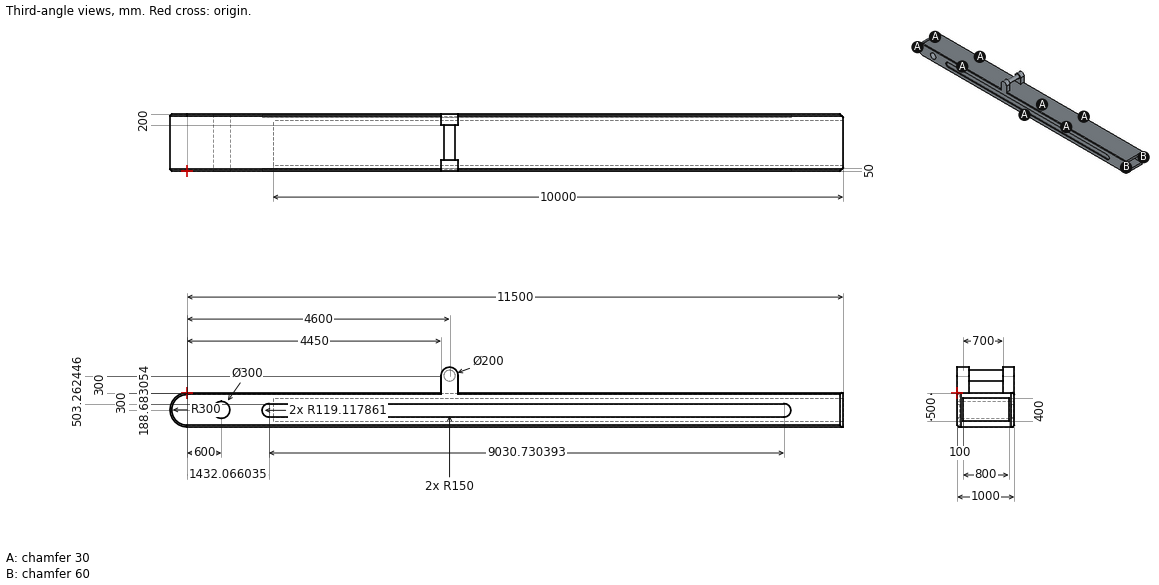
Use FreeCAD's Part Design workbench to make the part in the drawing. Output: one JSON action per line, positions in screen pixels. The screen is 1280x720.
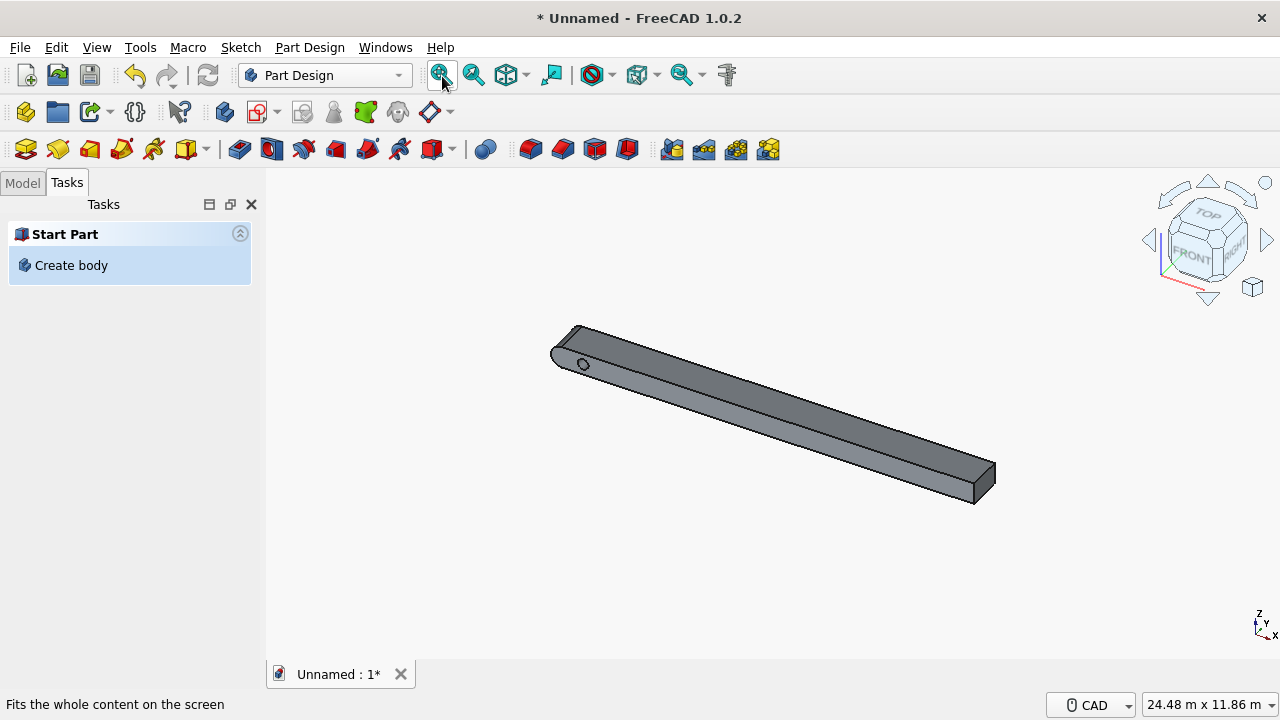
{"action": "key", "text": "4"}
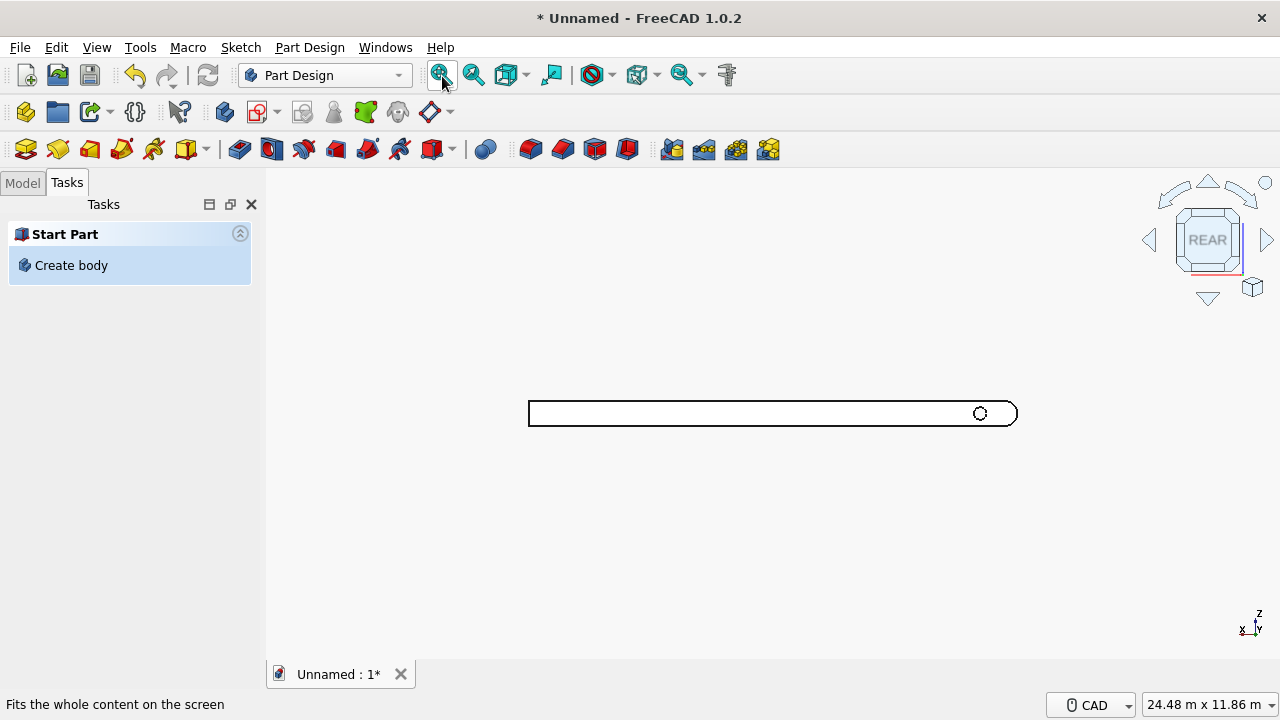
{"action": "left_click", "coordinate": [564, 412]}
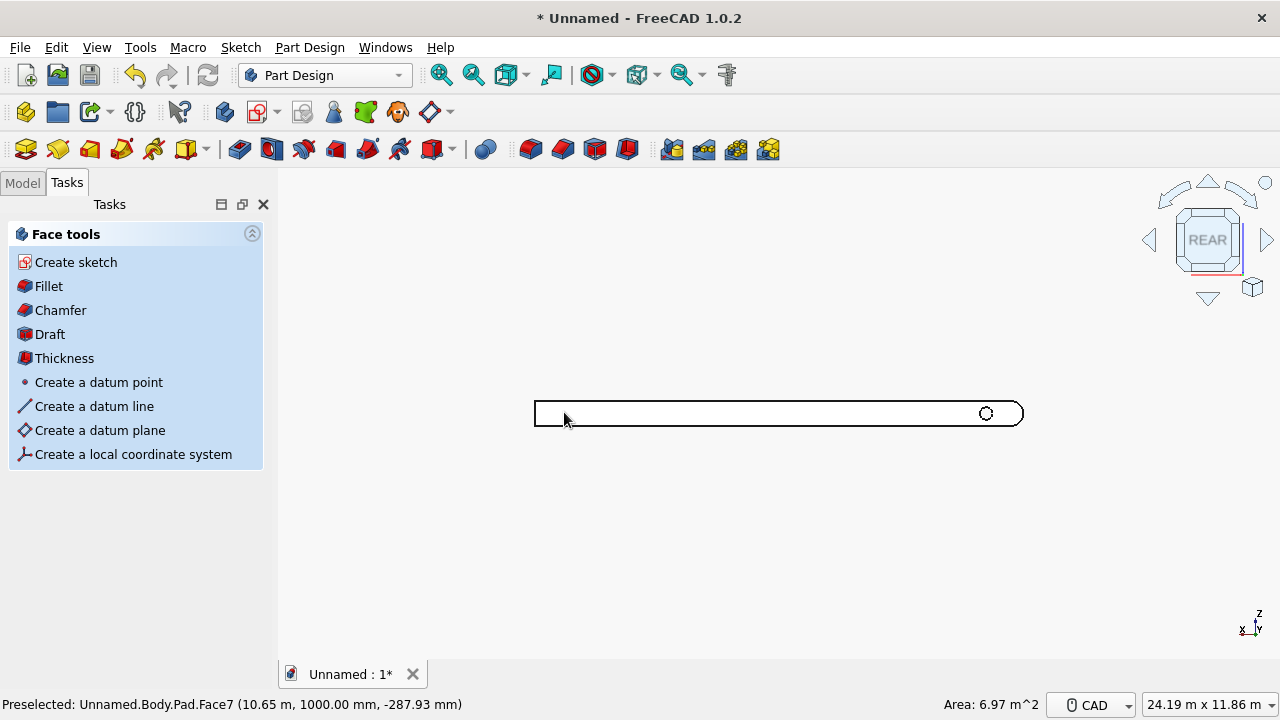
{"action": "left_click", "coordinate": [258, 112]}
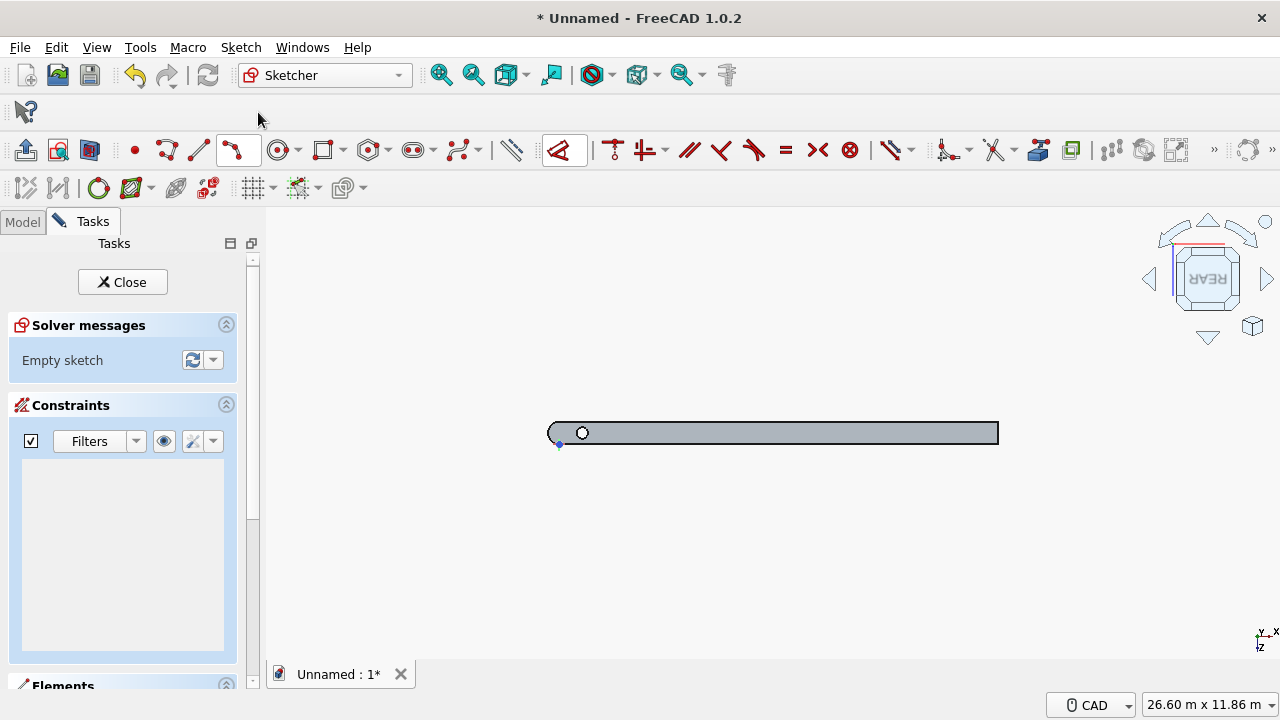
{"action": "scroll", "coordinate": [739, 448], "scroll_direction": "up", "scroll_amount": 11}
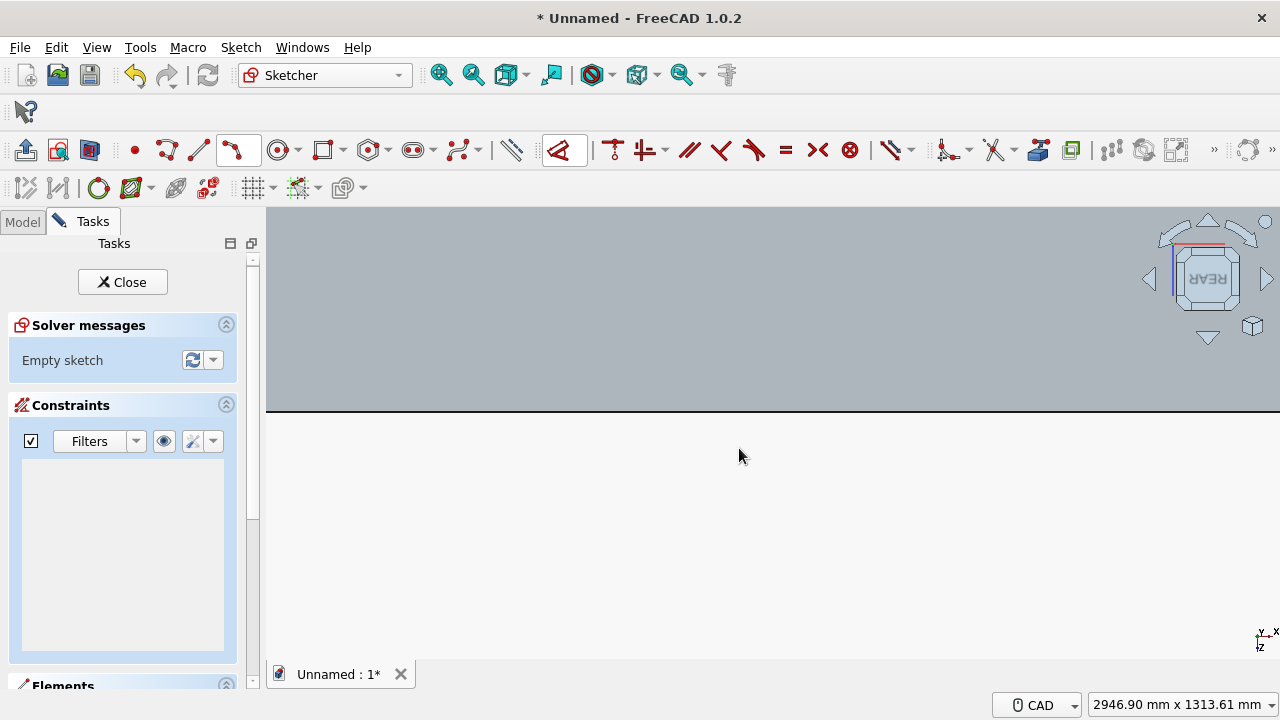
{"action": "left_click", "coordinate": [414, 150]}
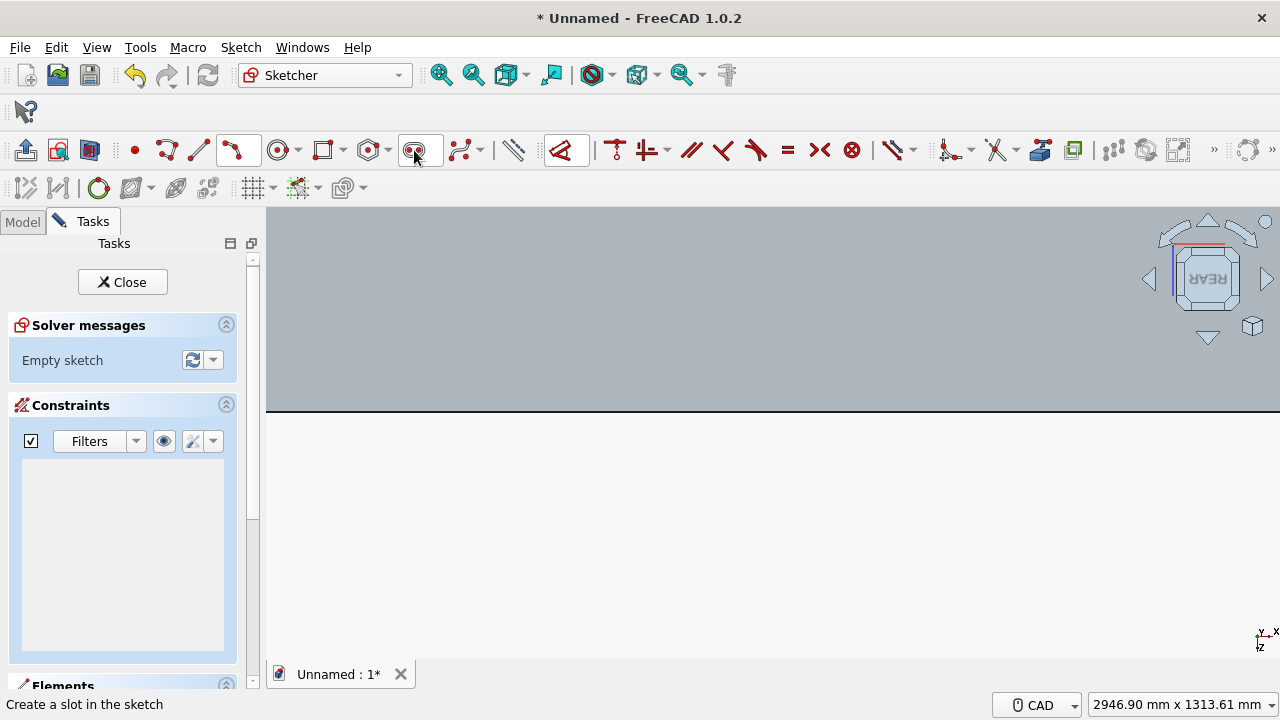
{"action": "left_click", "coordinate": [698, 515]}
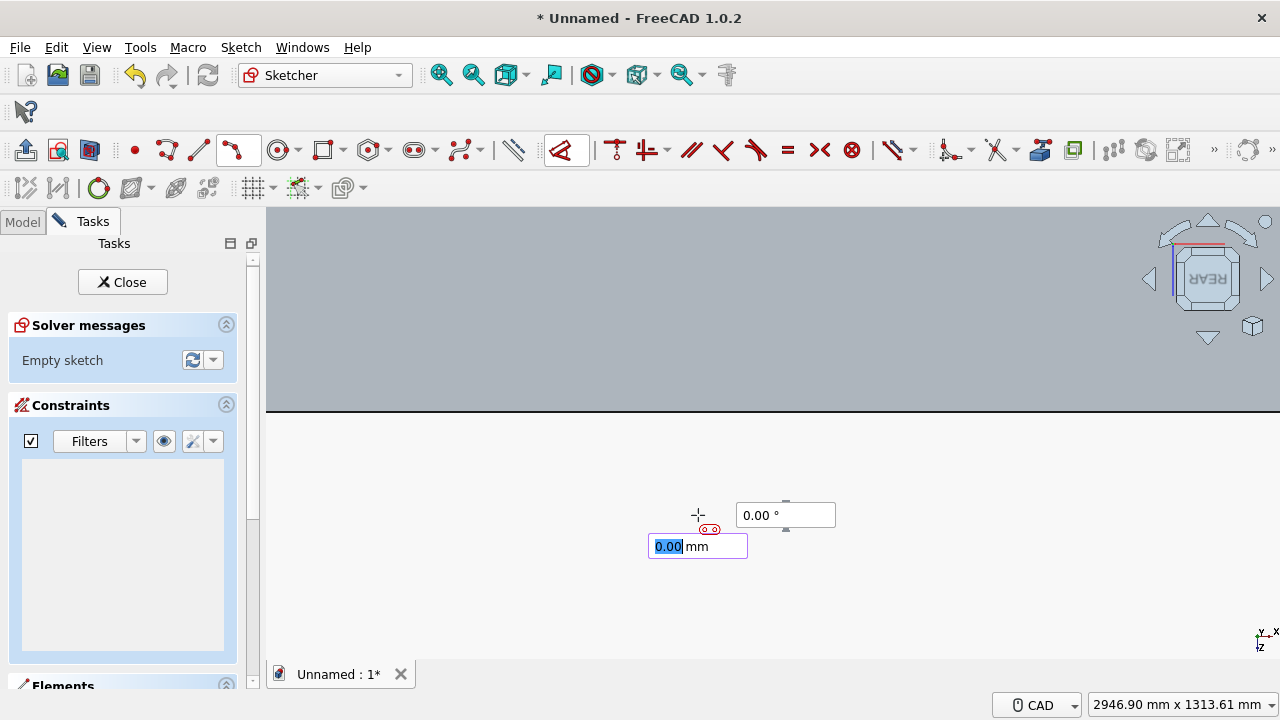
{"action": "left_click", "coordinate": [698, 342]}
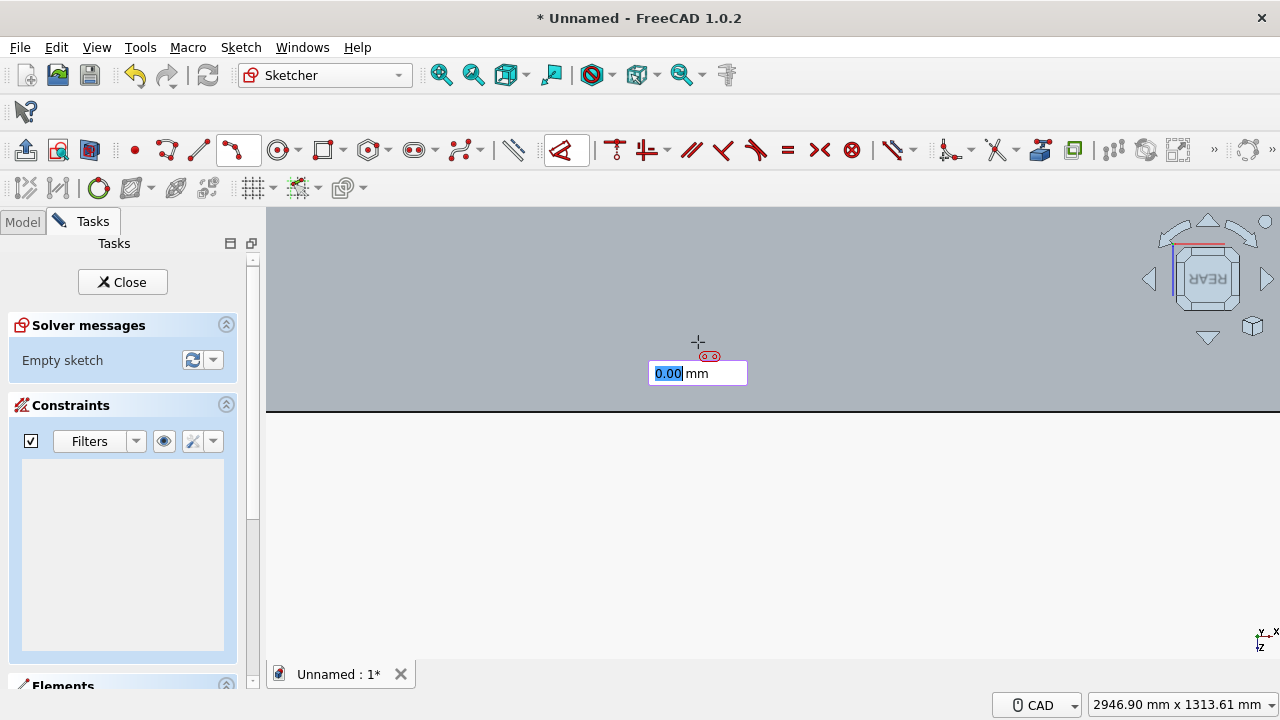
{"action": "left_click", "coordinate": [749, 428]}
{"action": "key", "text": "Escape"}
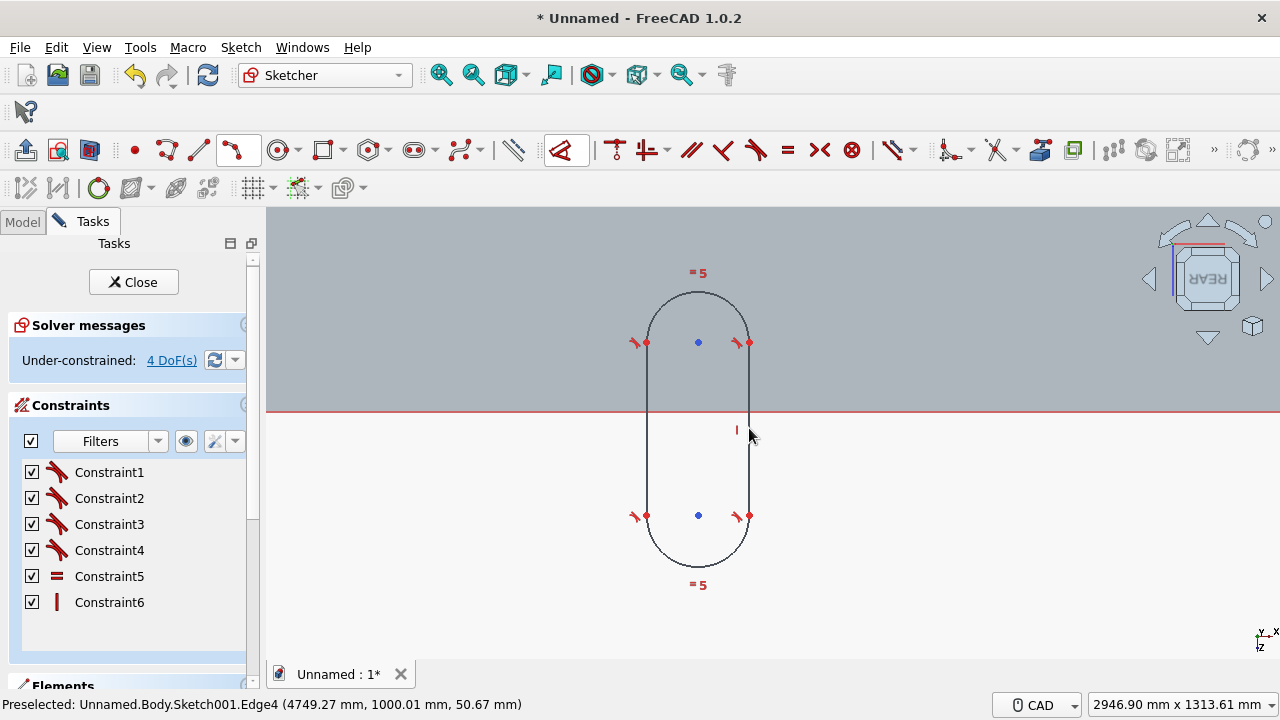
{"action": "left_click", "coordinate": [668, 557]}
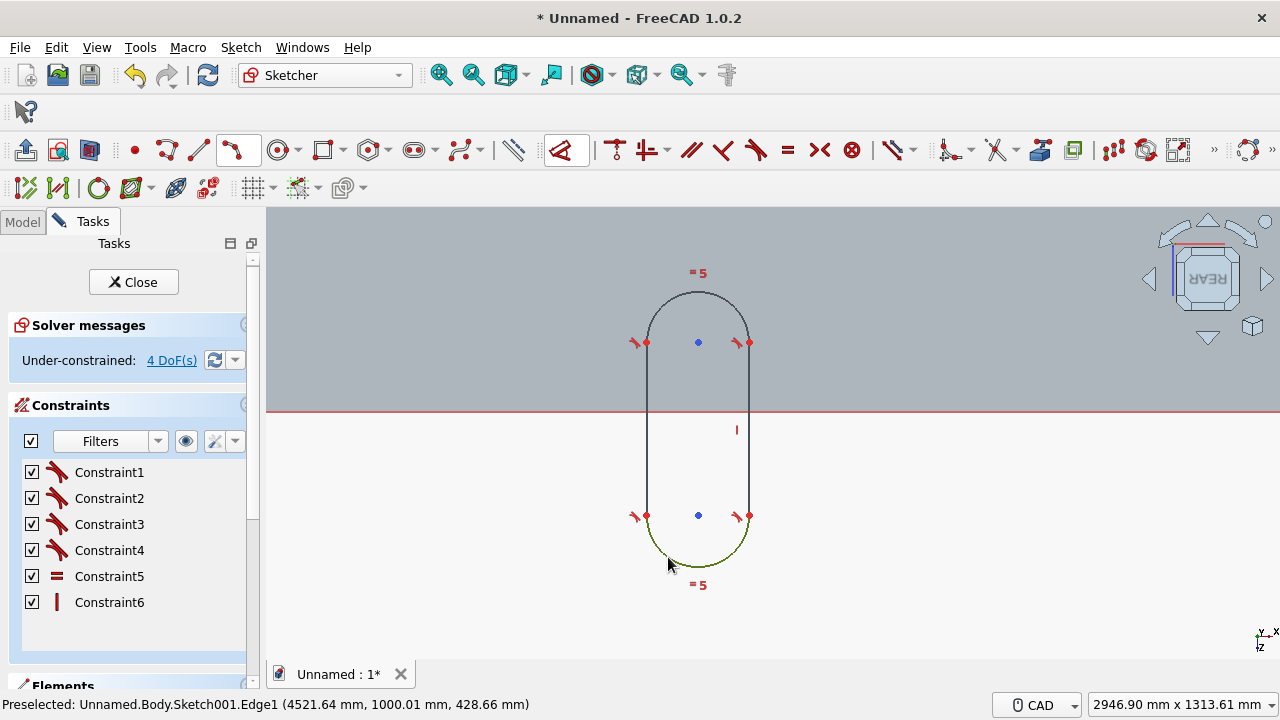
{"action": "left_click", "coordinate": [584, 150]}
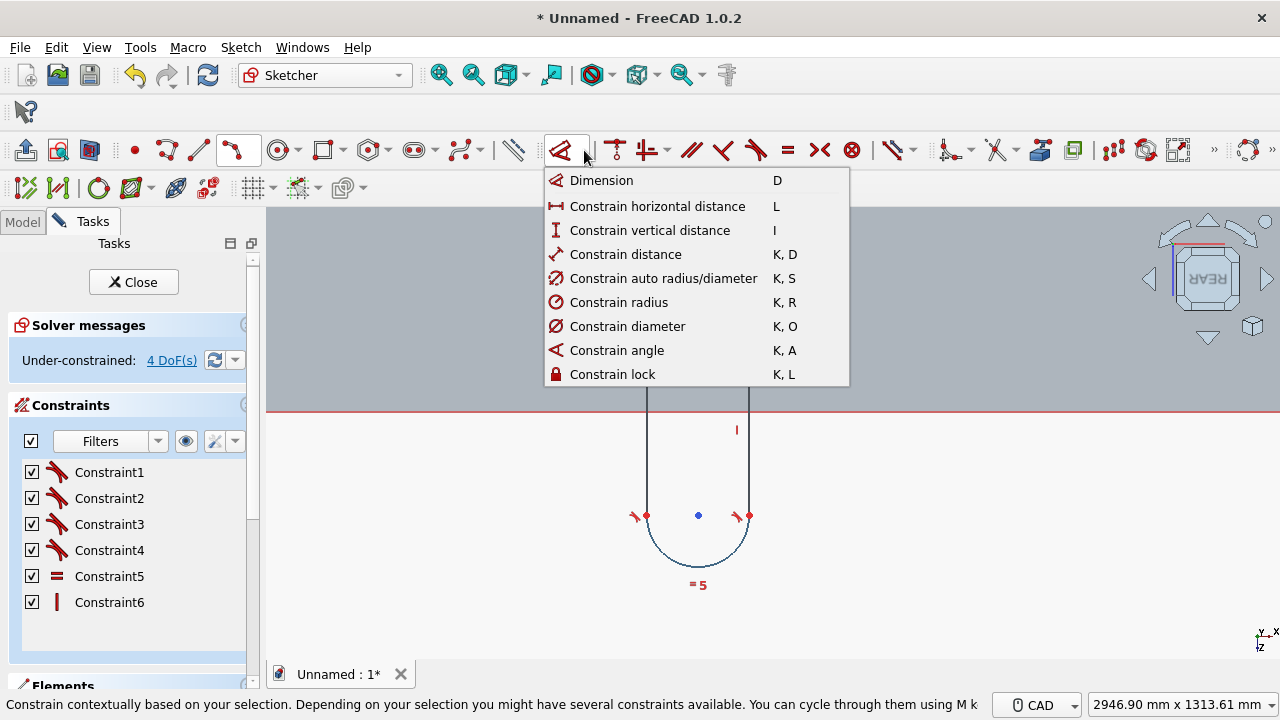
{"action": "left_click", "coordinate": [697, 302]}